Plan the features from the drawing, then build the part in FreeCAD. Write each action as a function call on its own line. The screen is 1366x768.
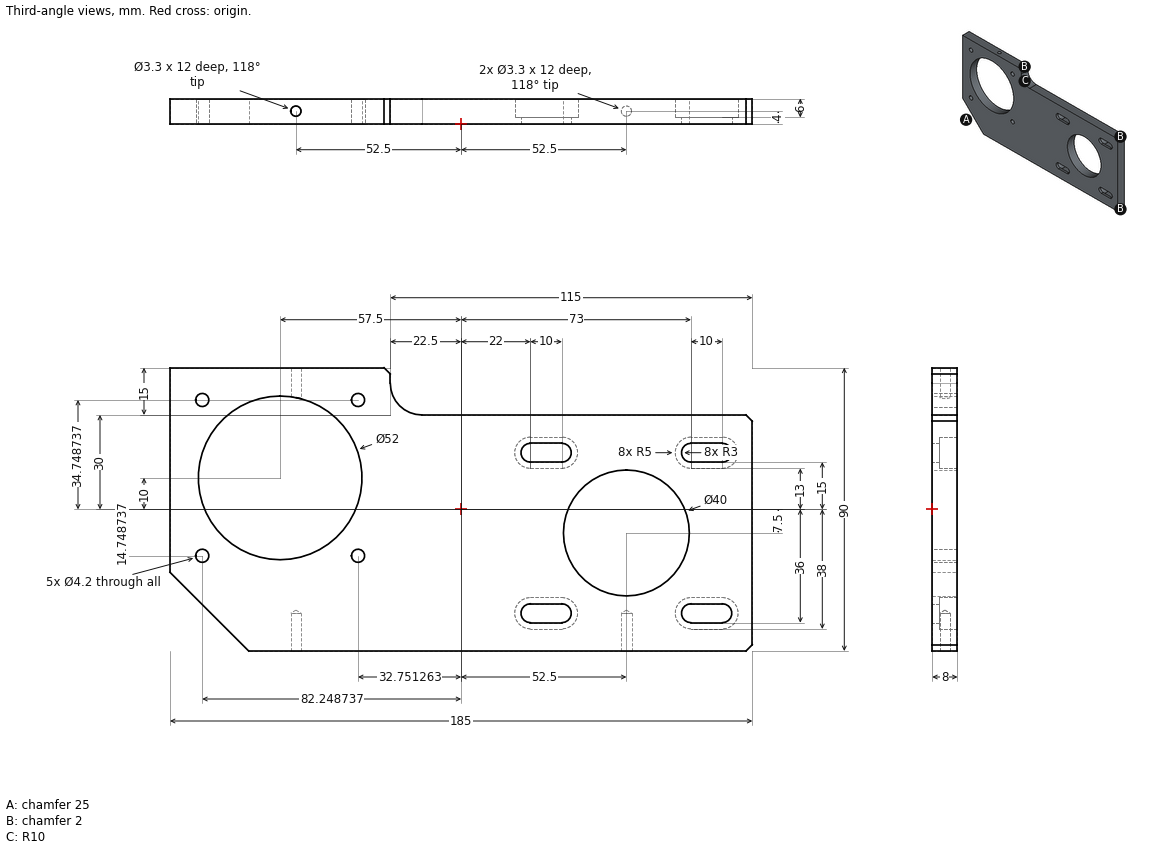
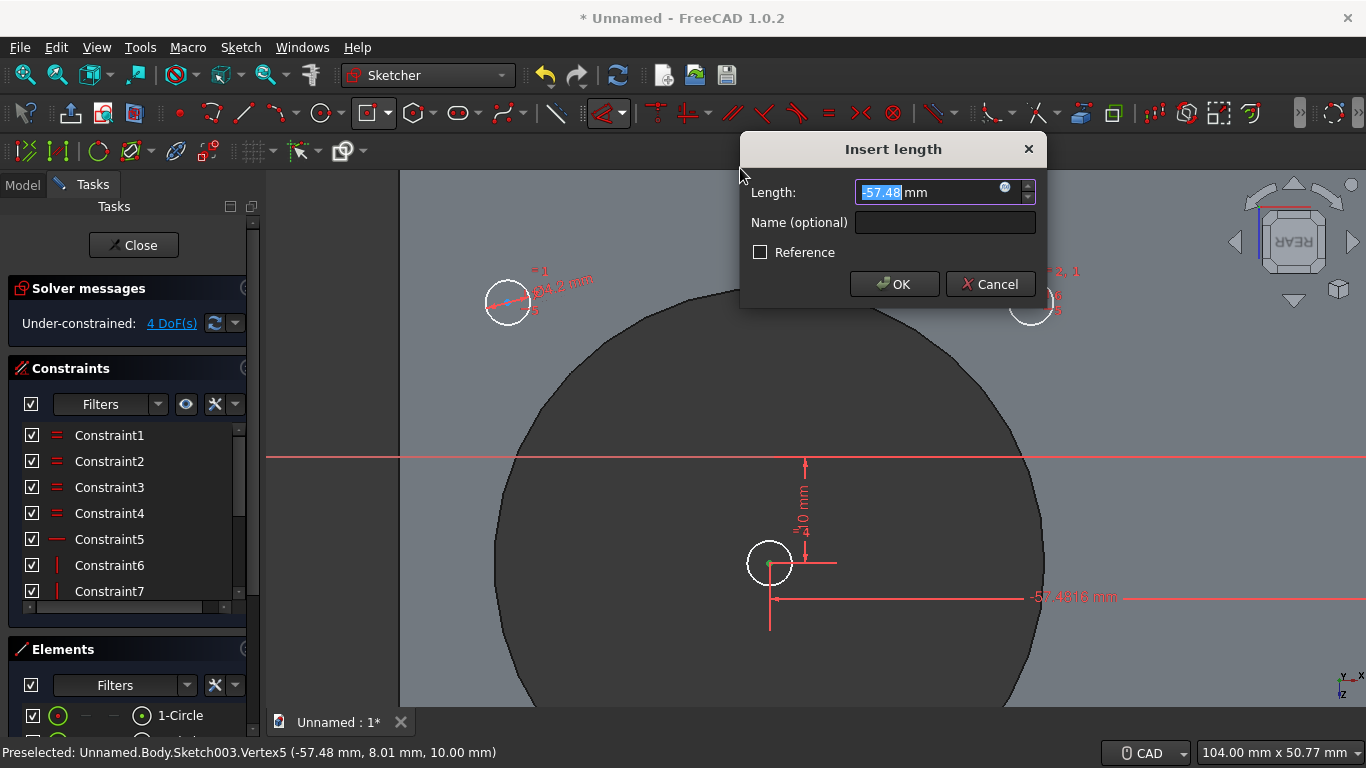
text(-57.5)
key(Return)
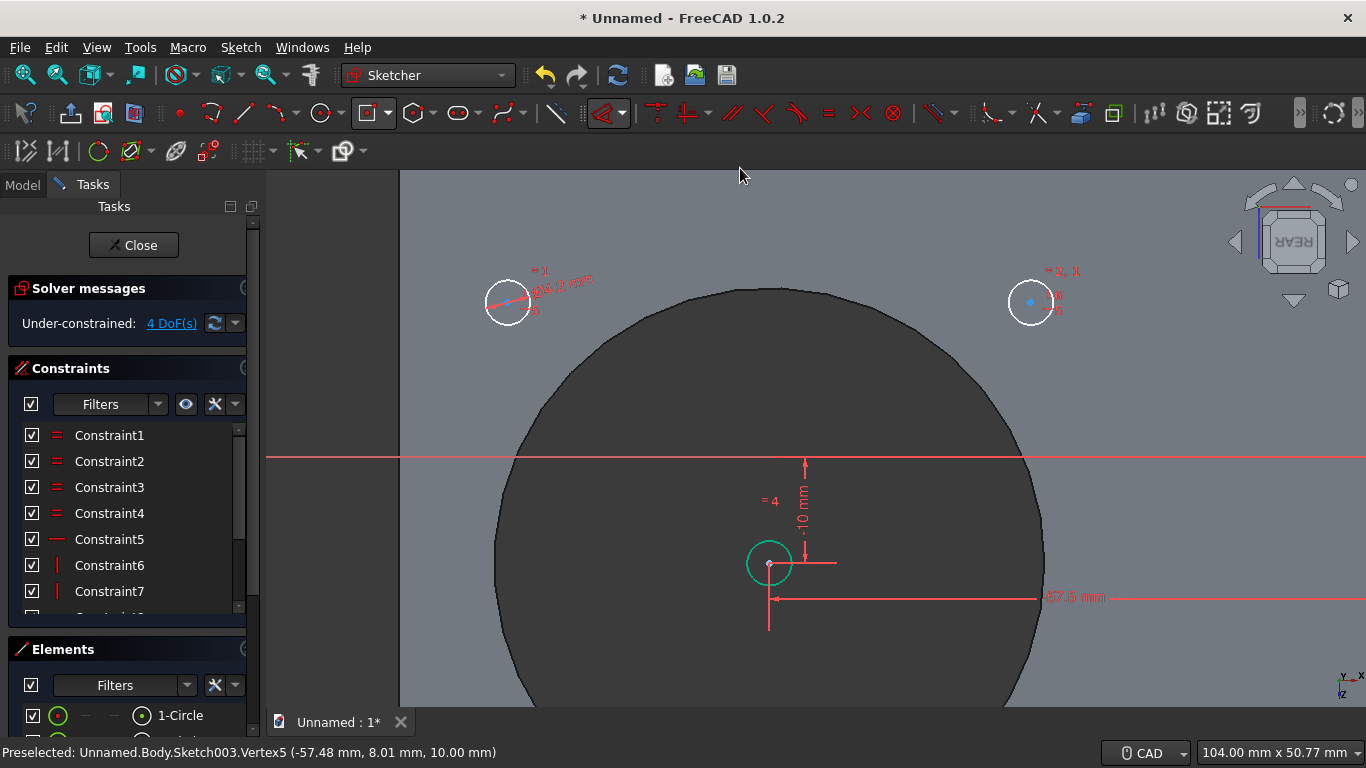
click(508, 303)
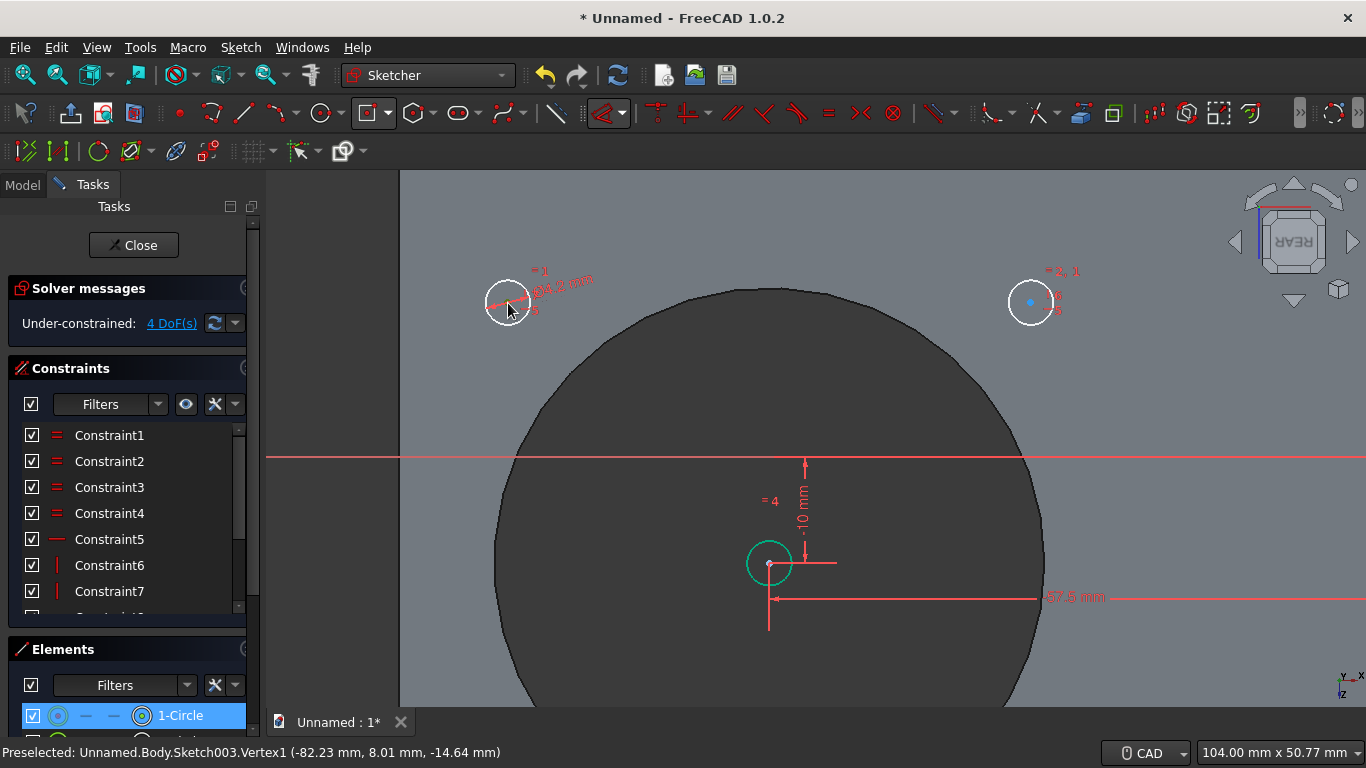
key(l)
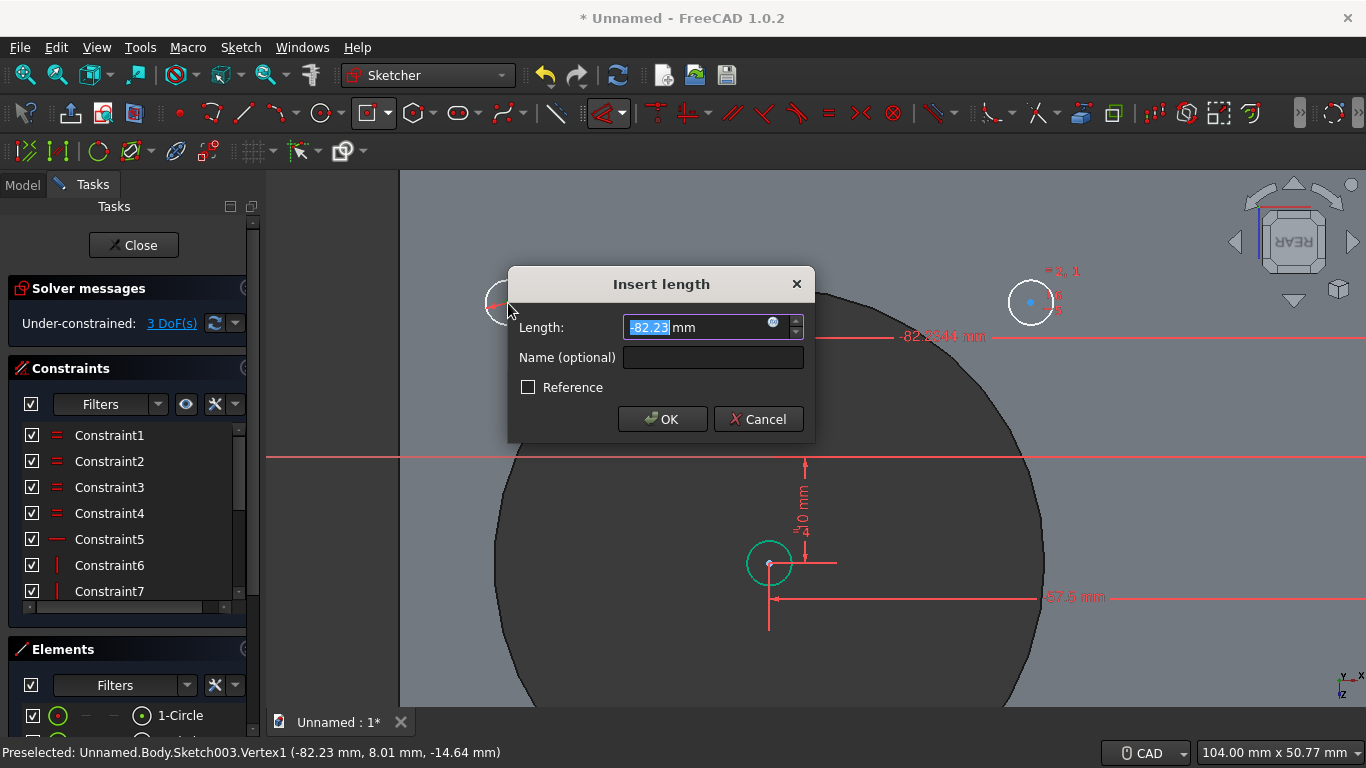
text(-82.248737)
key(Return)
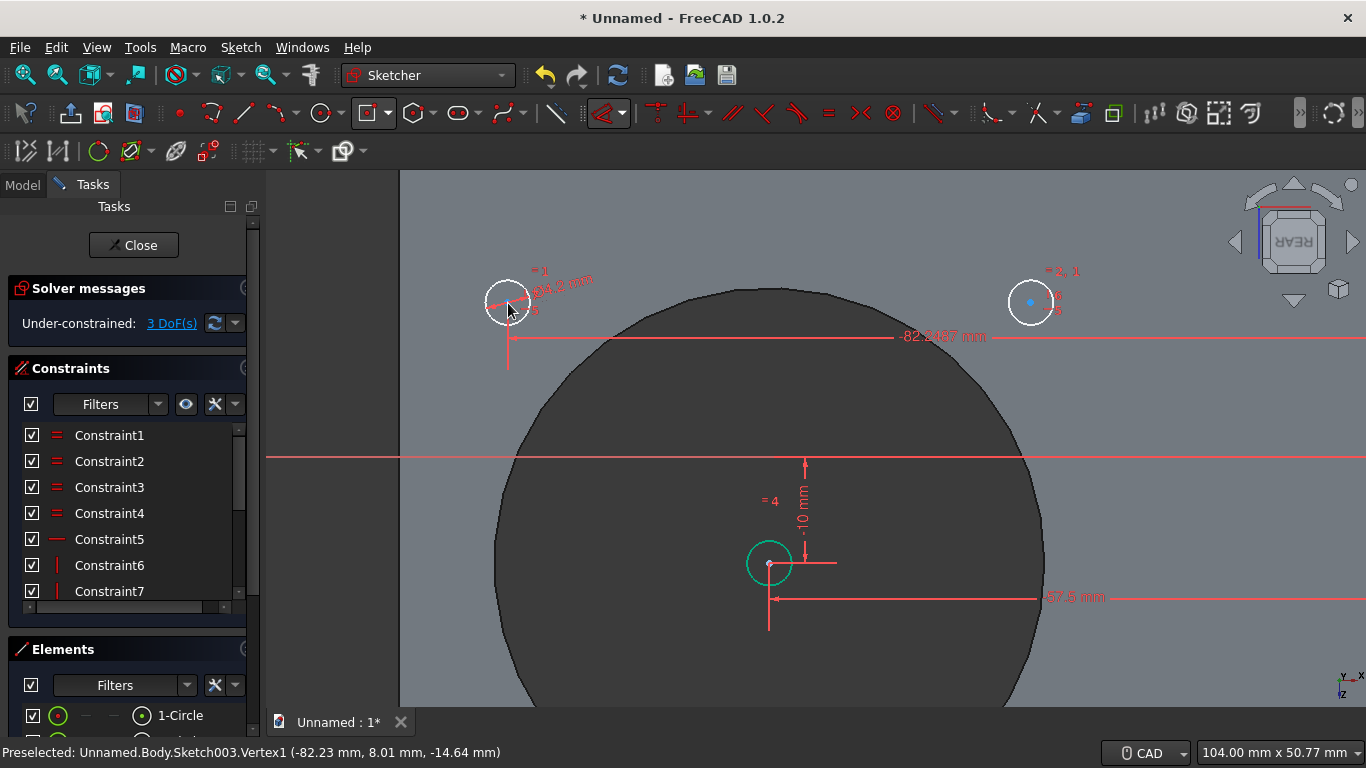
click(508, 303)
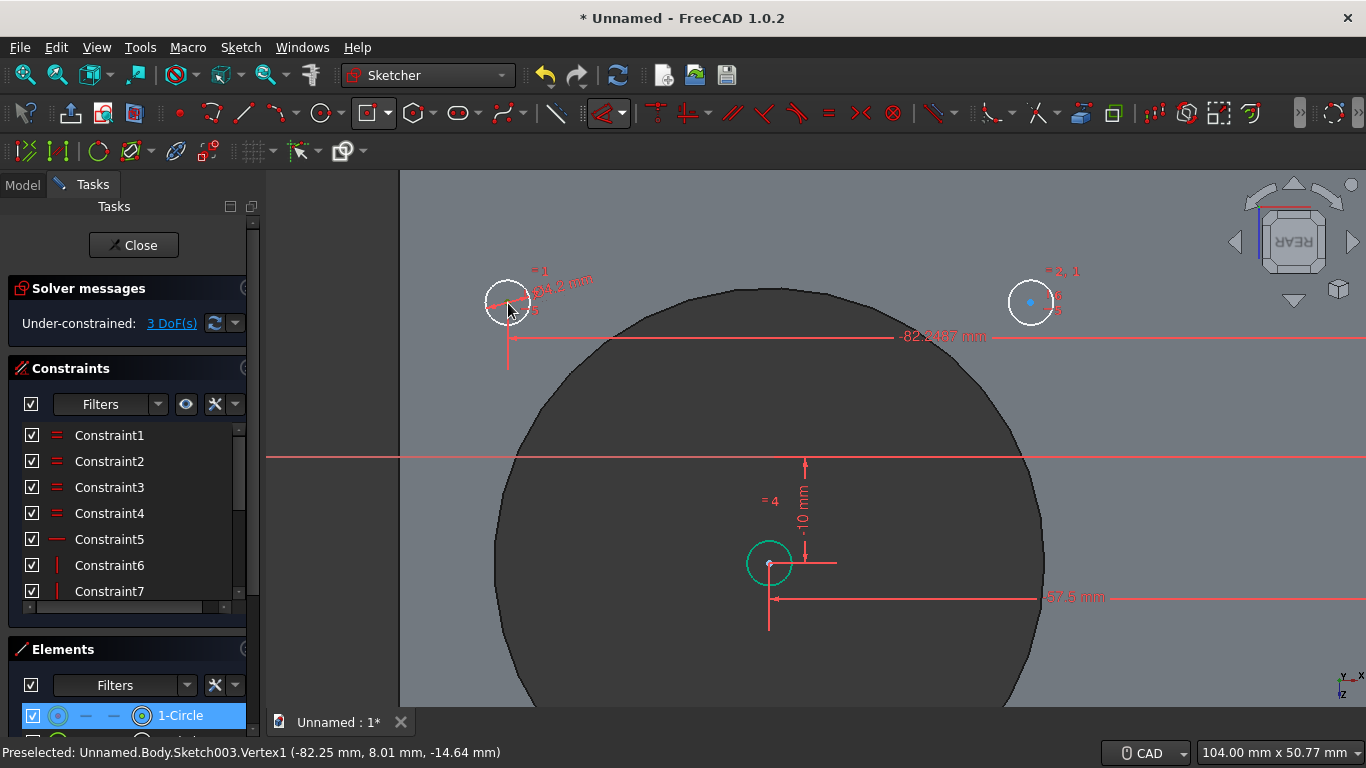
key(i)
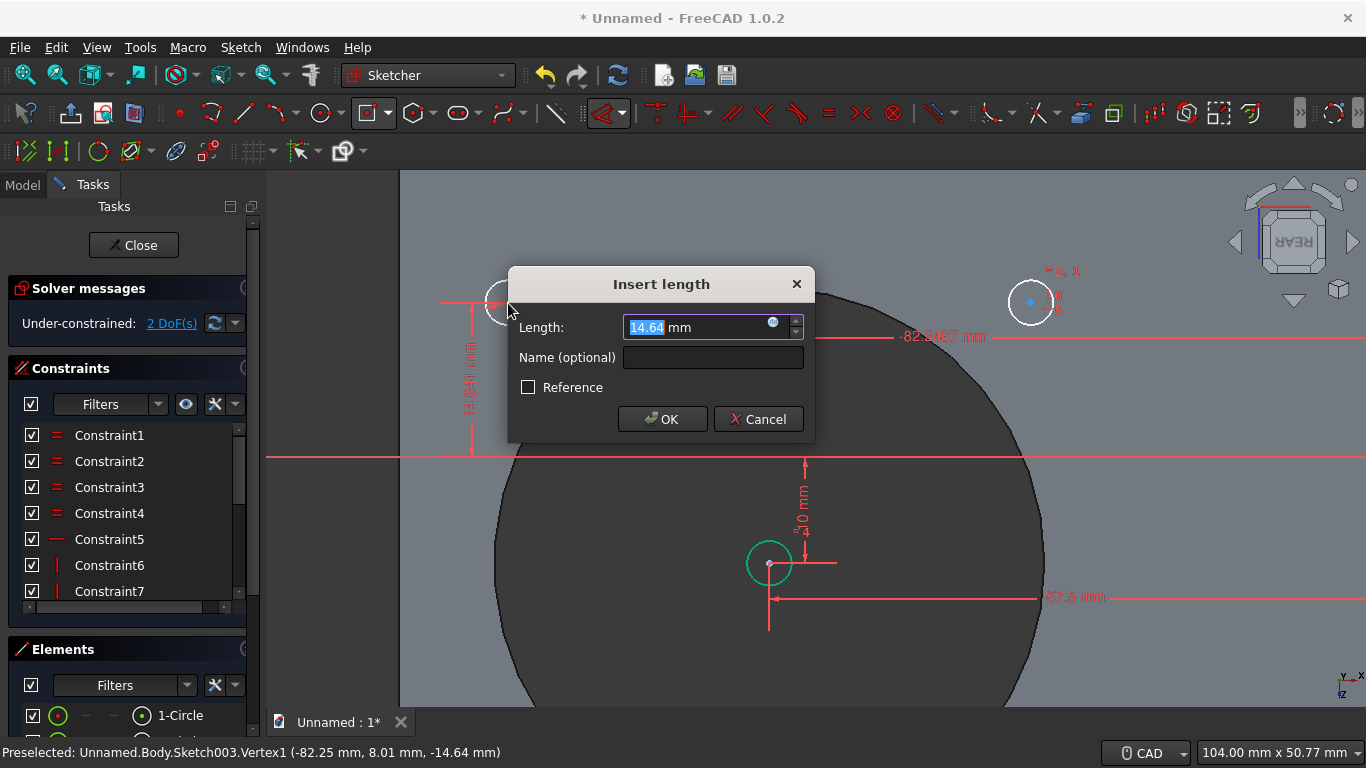
text(14.748737)
key(Return)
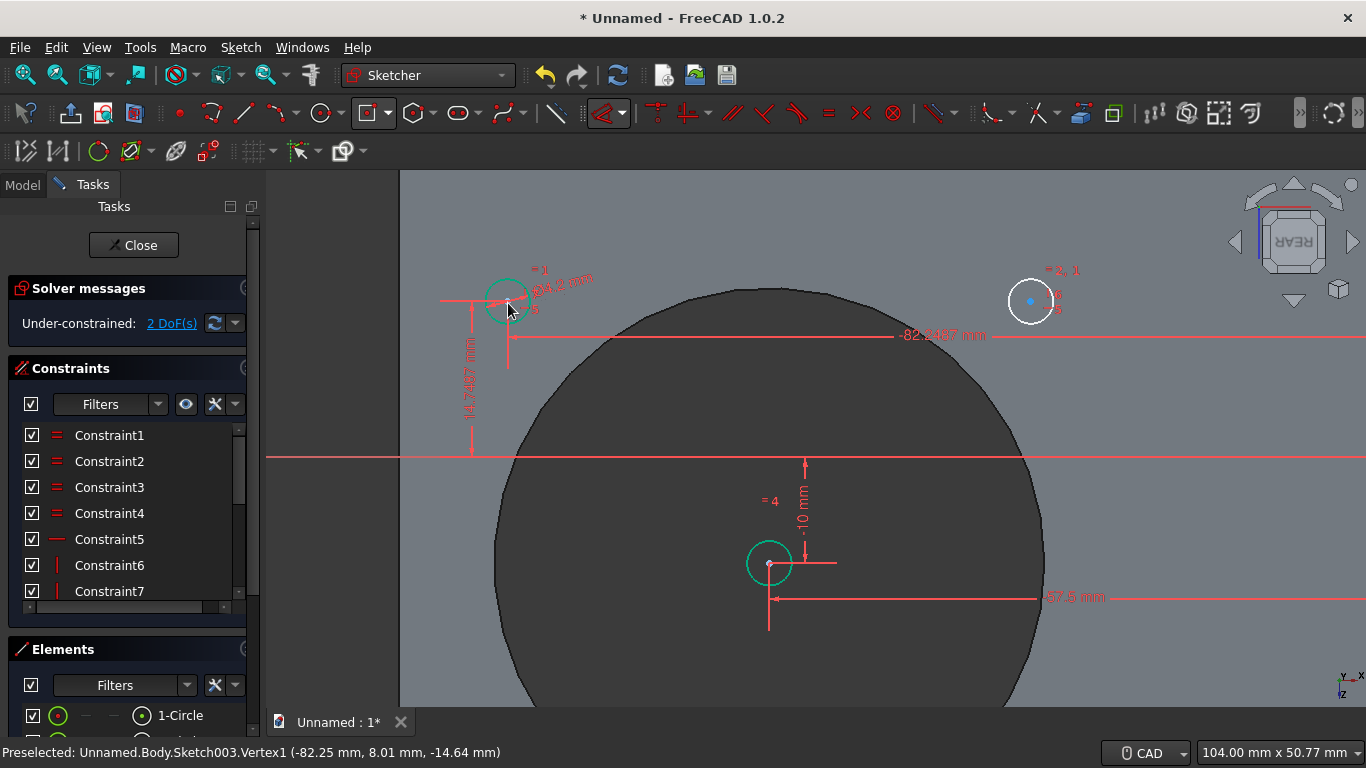
click(1031, 301)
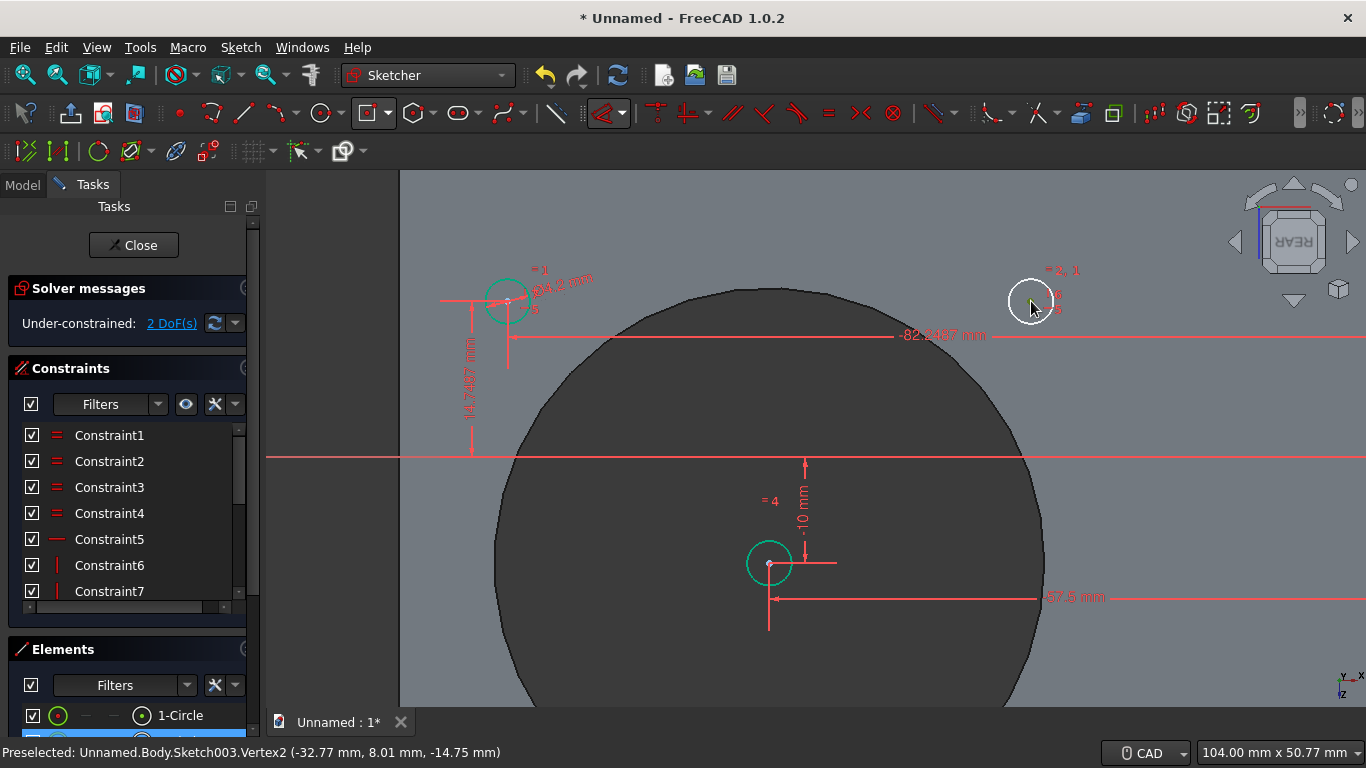
click(624, 114)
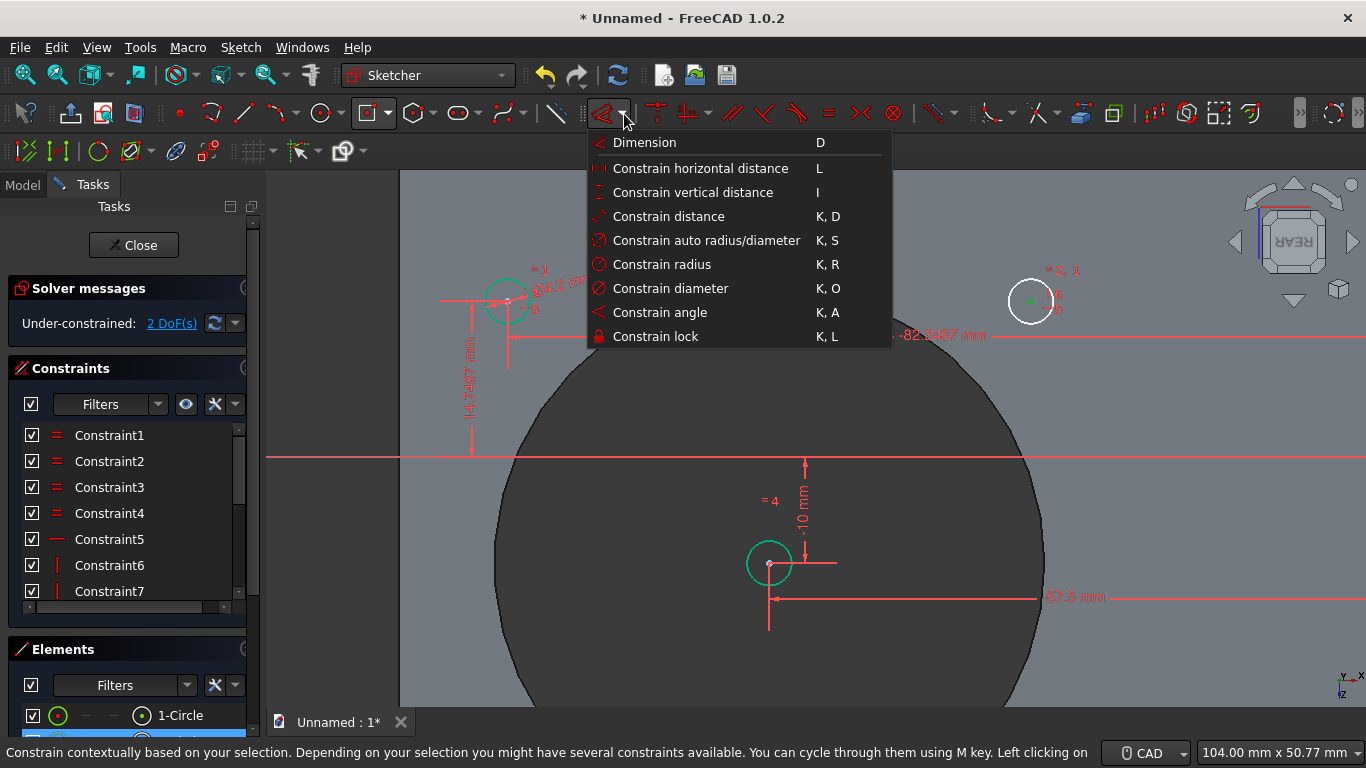
click(740, 168)